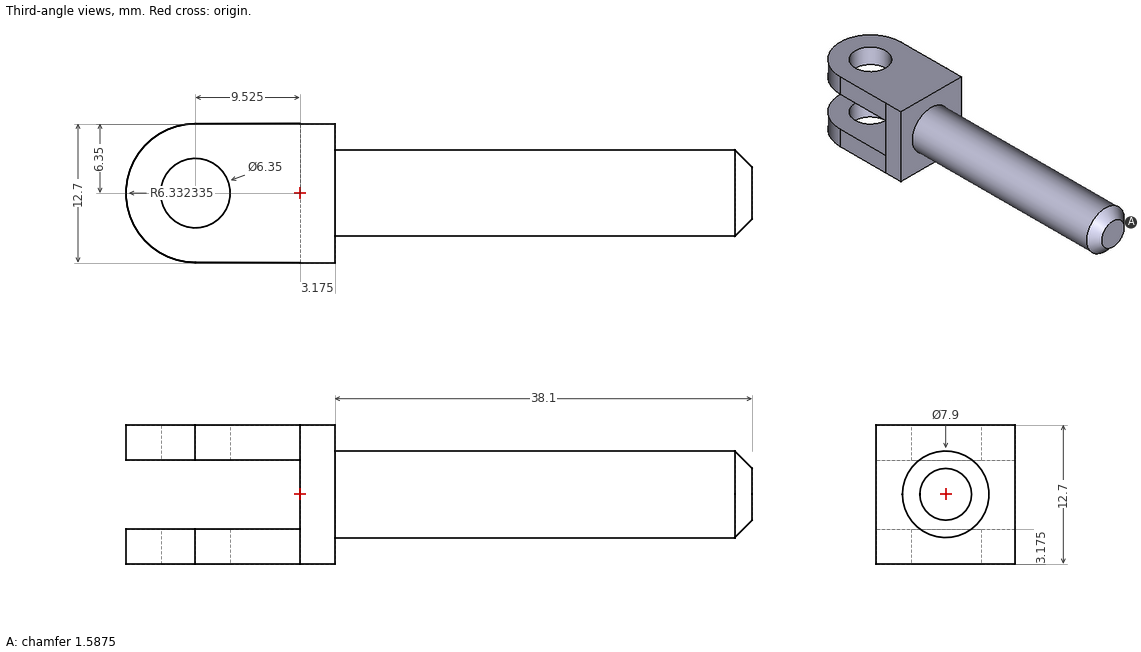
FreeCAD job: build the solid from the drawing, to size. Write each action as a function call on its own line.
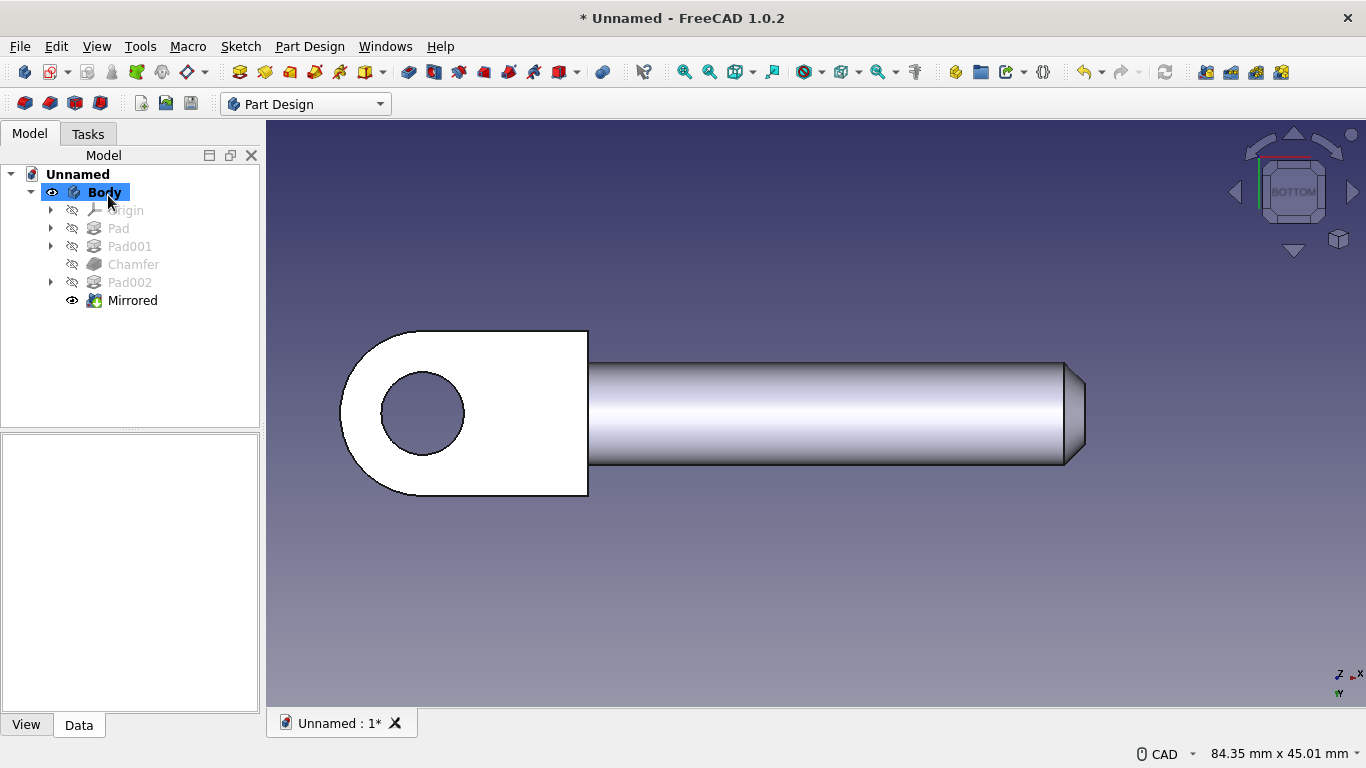
key(0)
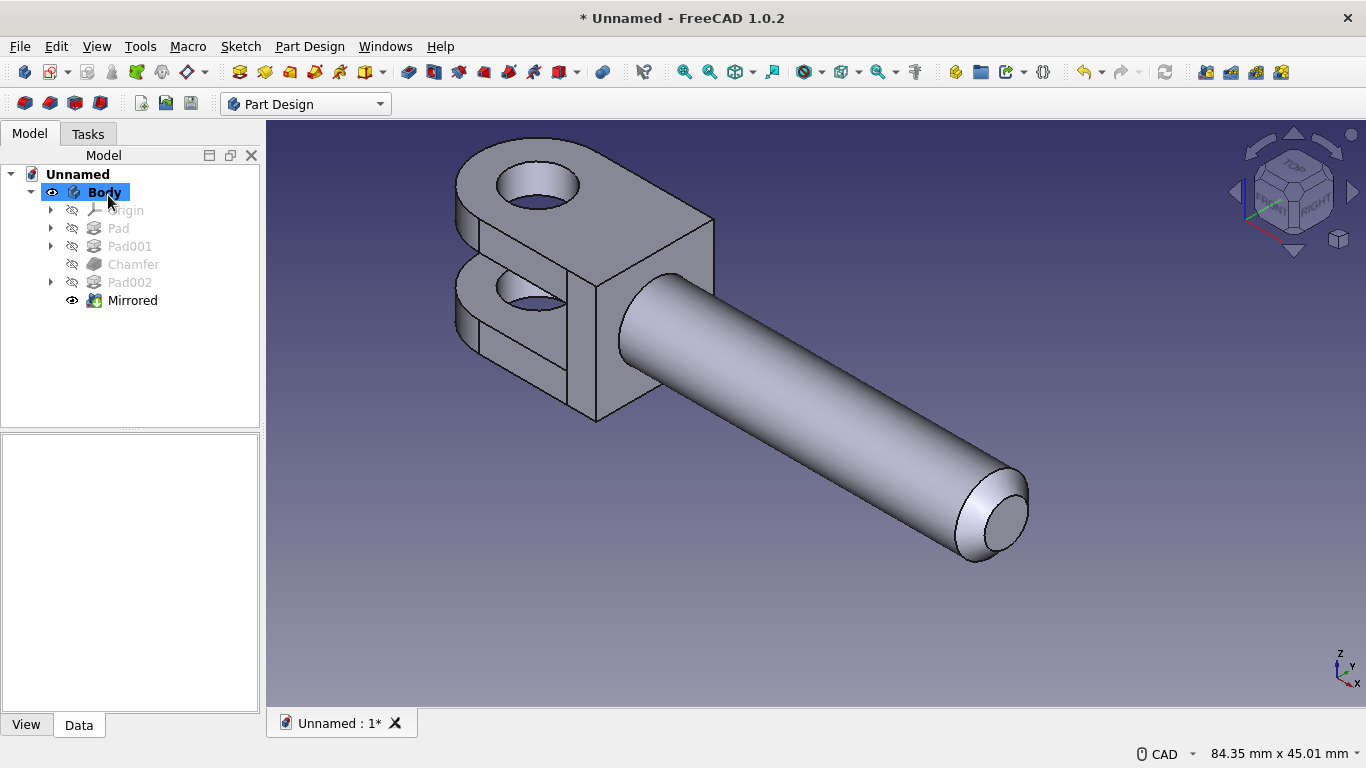
click(685, 72)